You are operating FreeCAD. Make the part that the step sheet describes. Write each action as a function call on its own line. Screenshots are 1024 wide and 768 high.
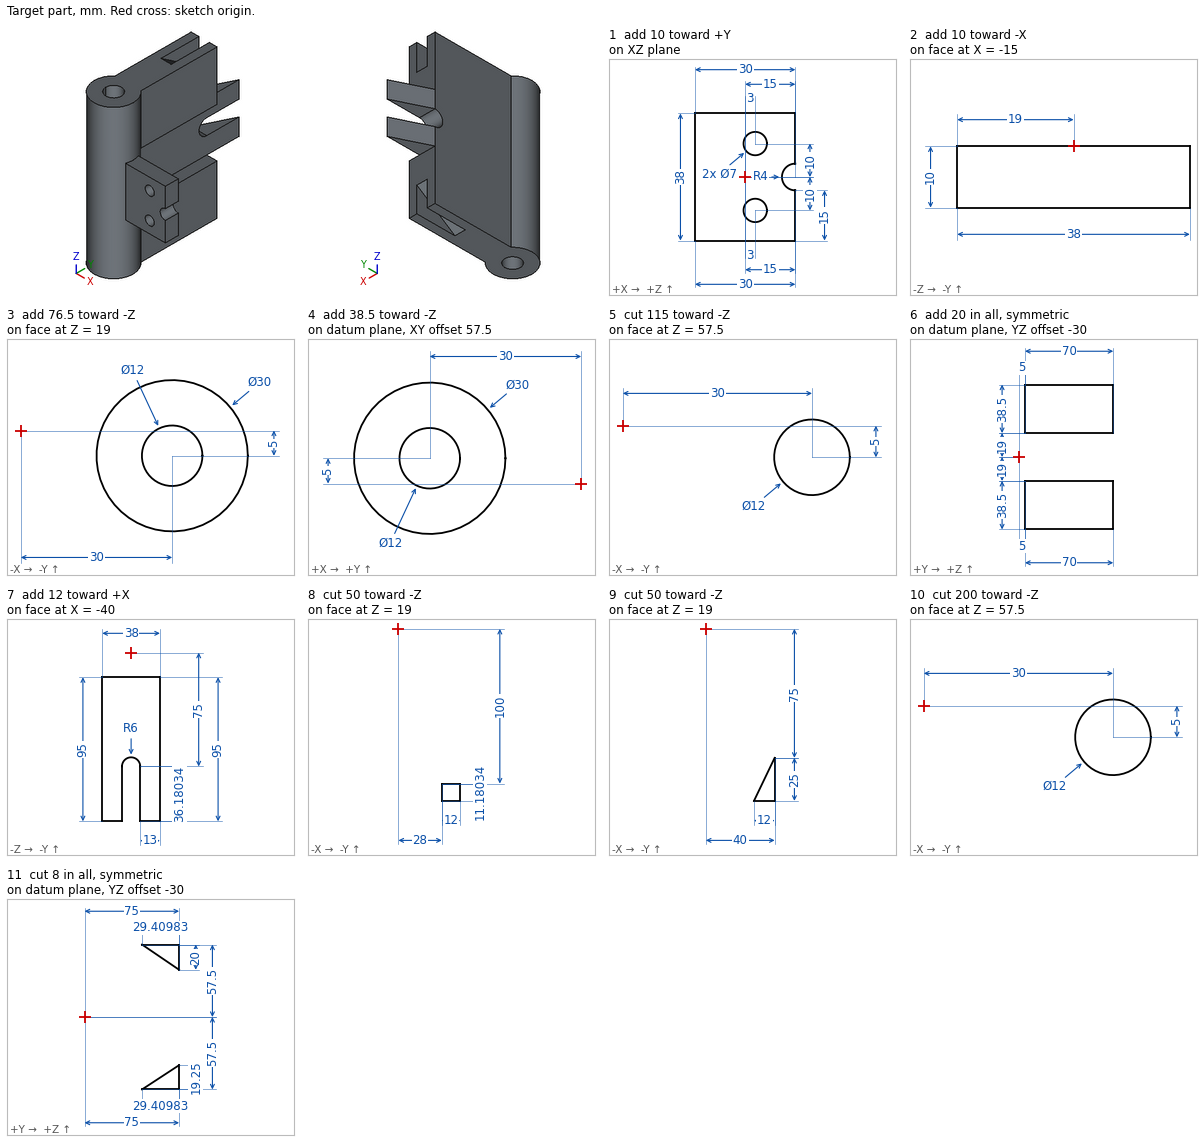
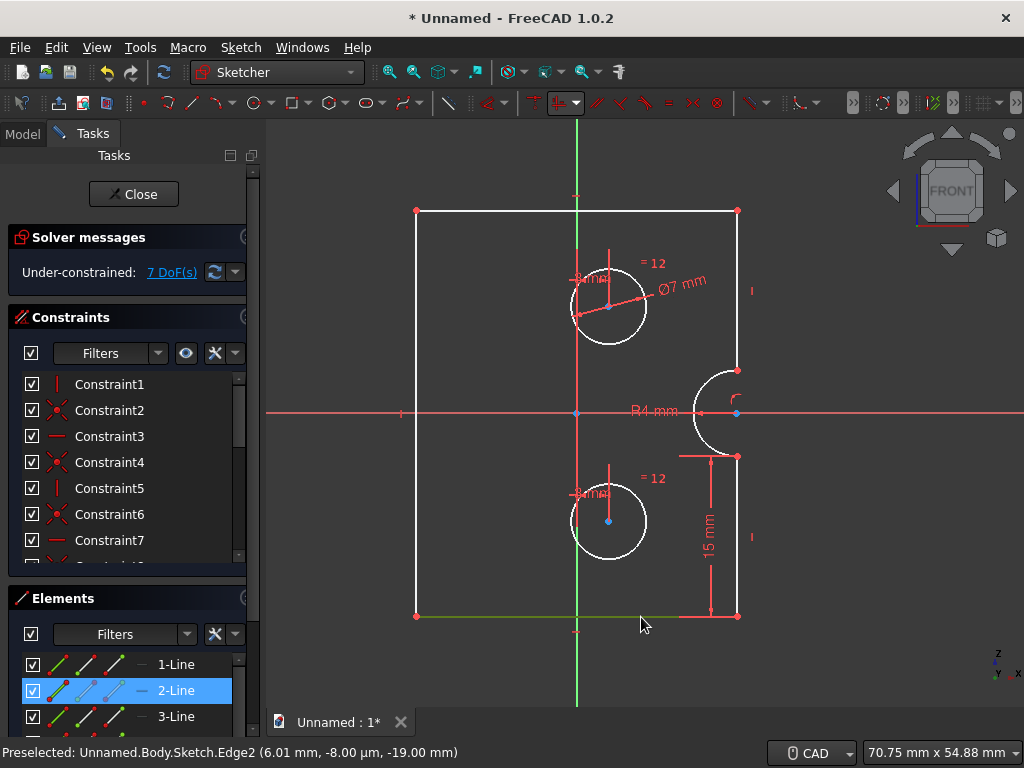
click(506, 104)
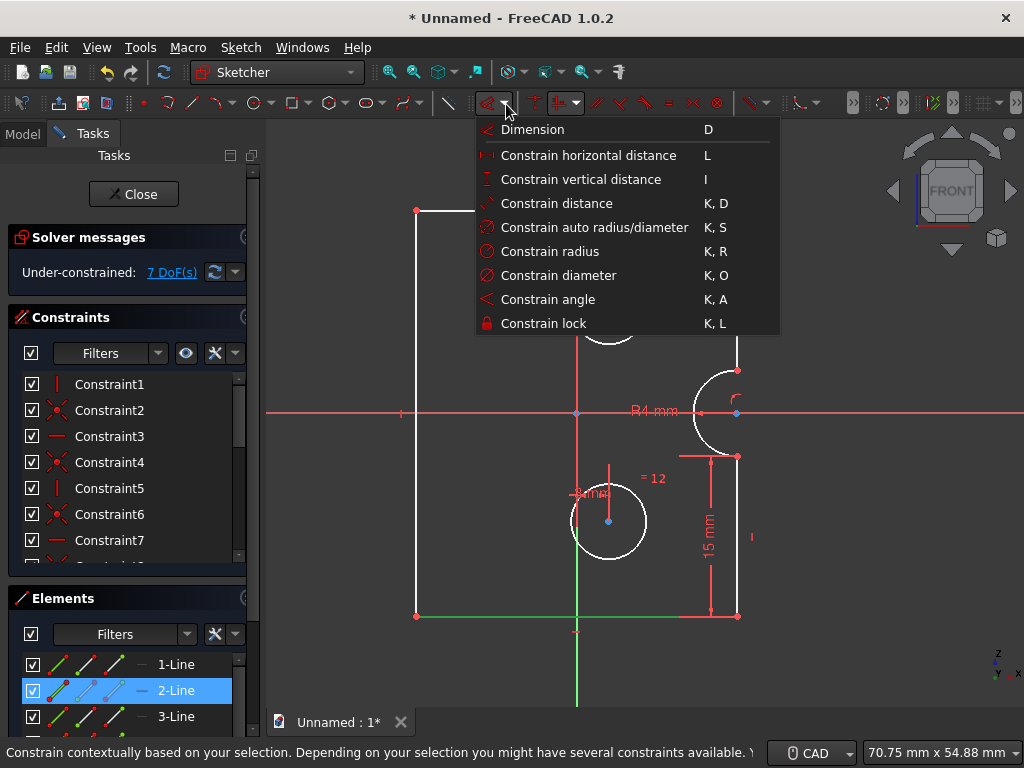
click(628, 155)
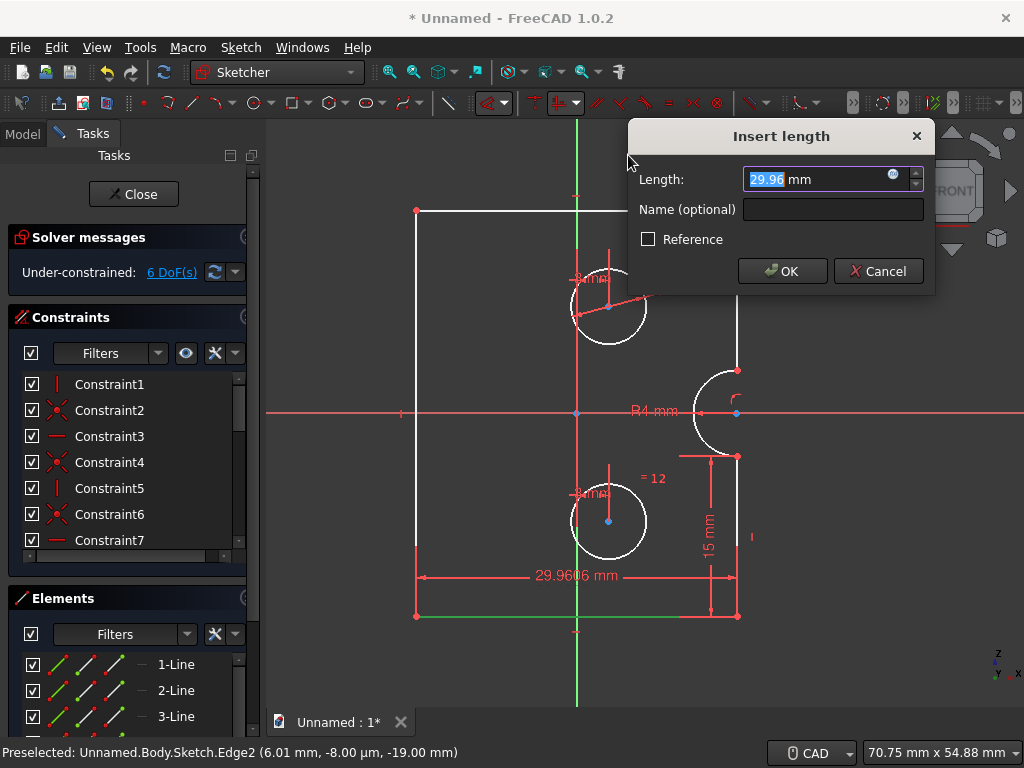
text(30)
key(Return)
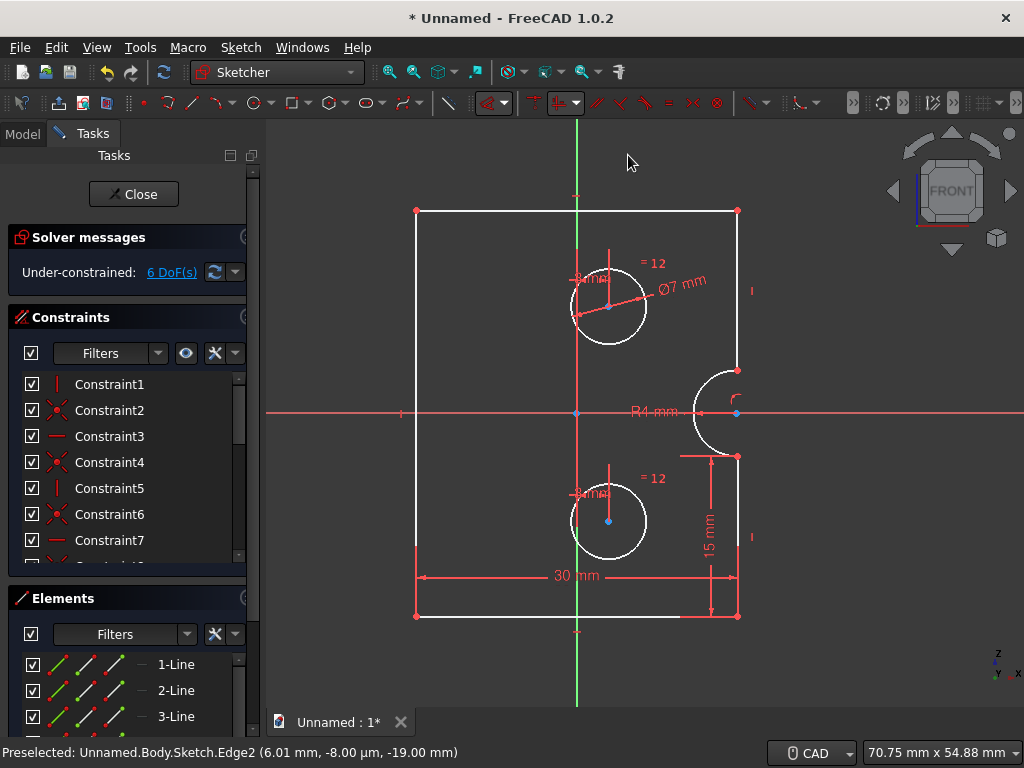
click(416, 495)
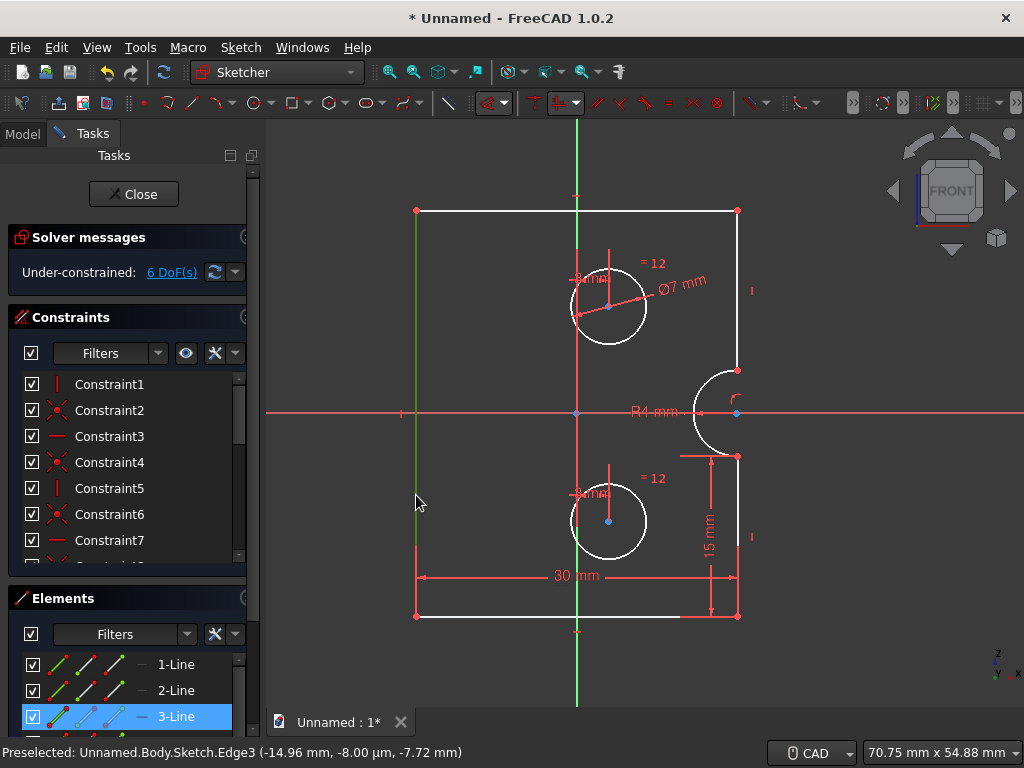
click(506, 104)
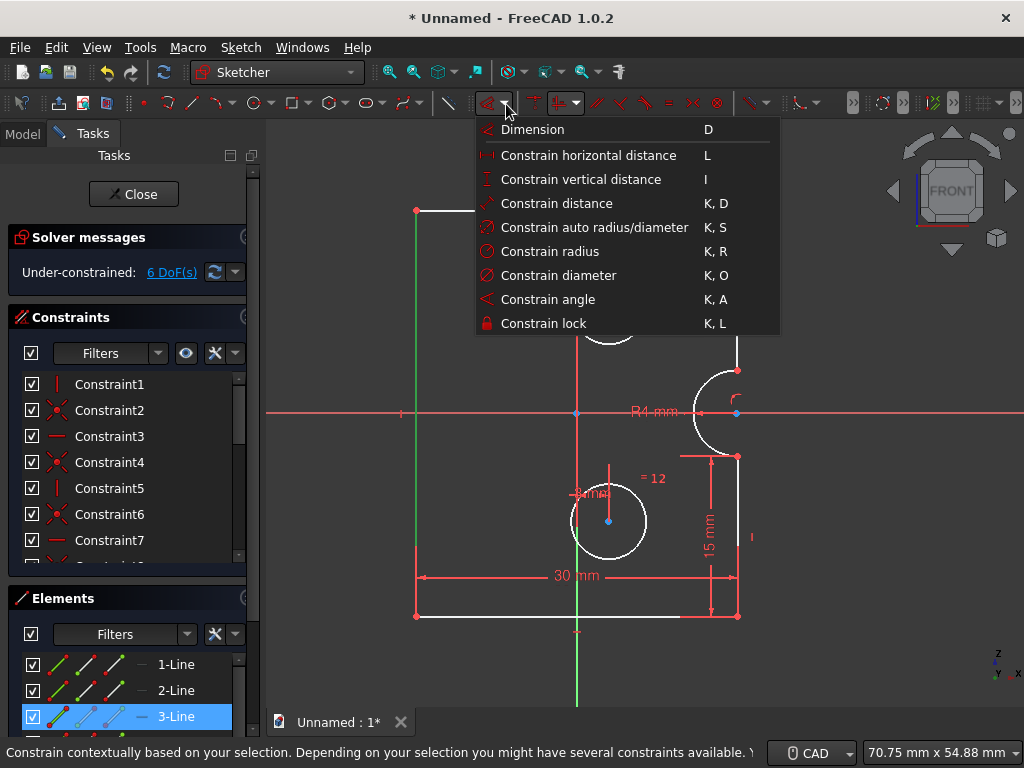
click(628, 179)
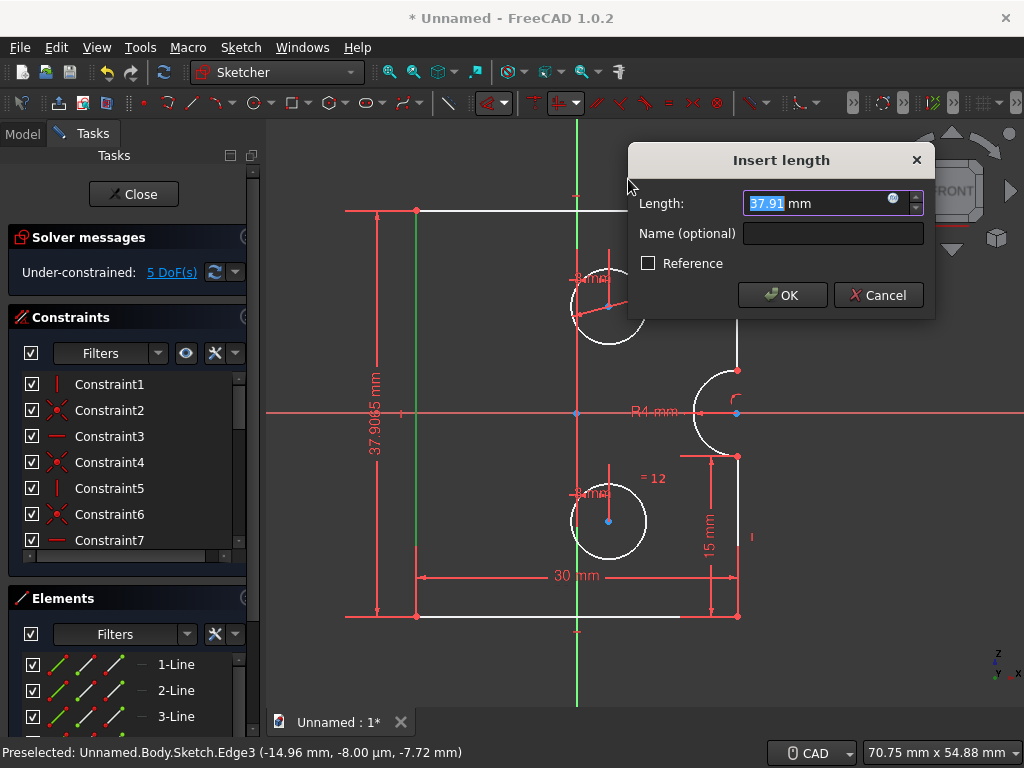
text(38)
key(Return)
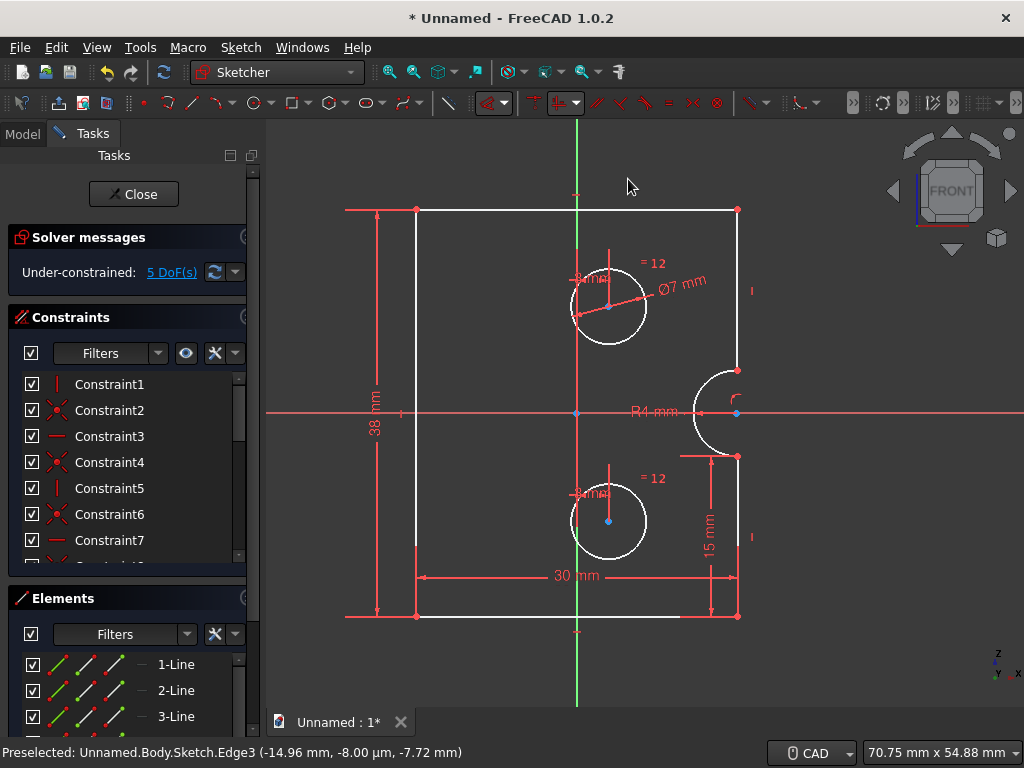
click(513, 210)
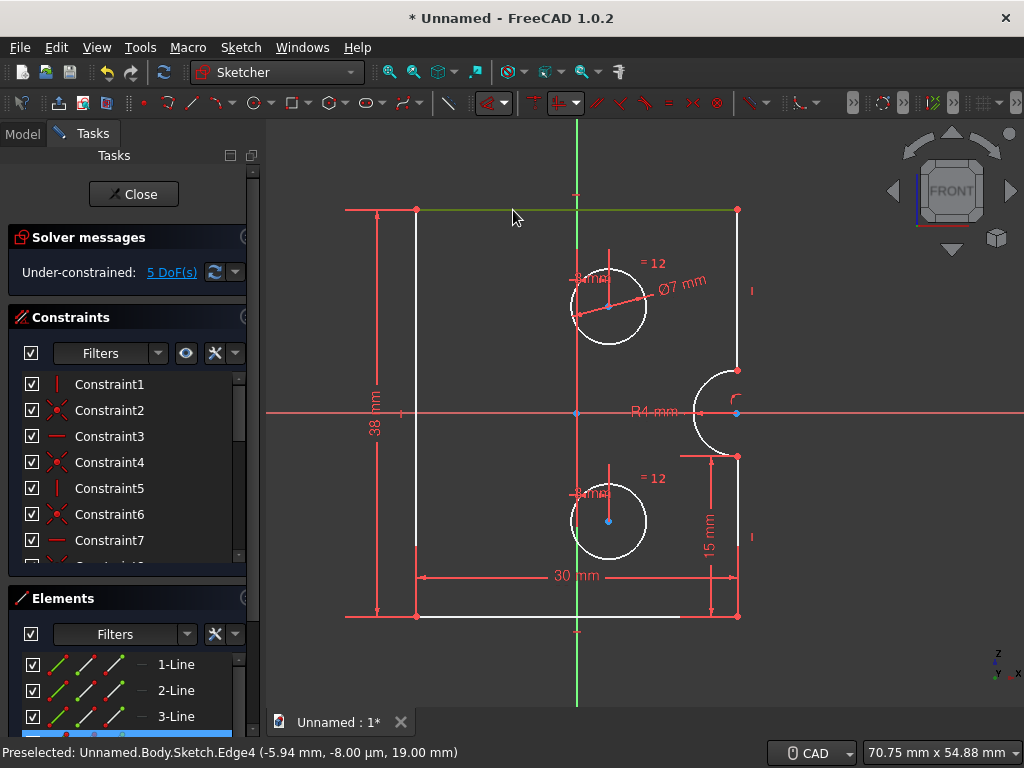
click(506, 104)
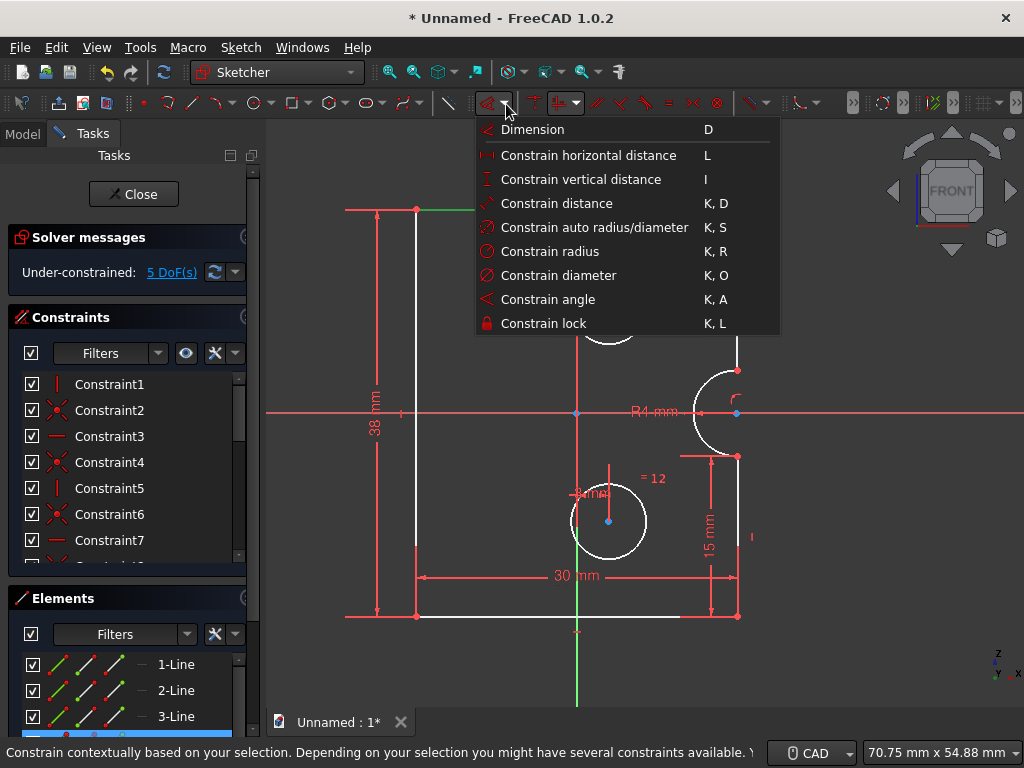
click(628, 155)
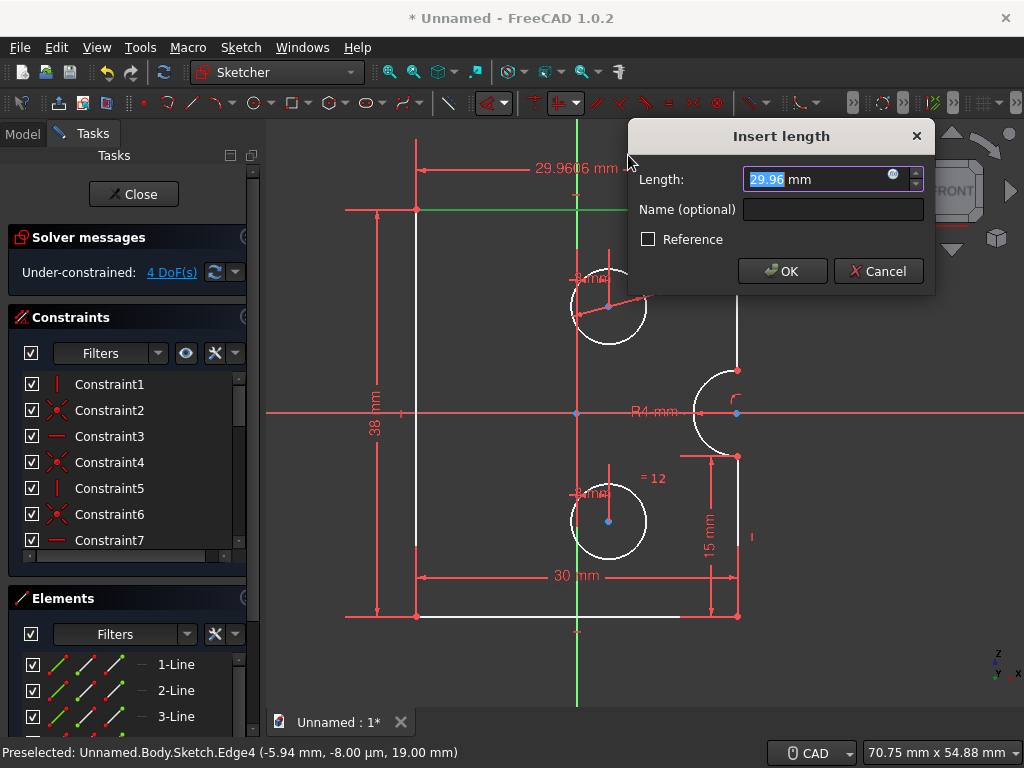
text(30)
key(Return)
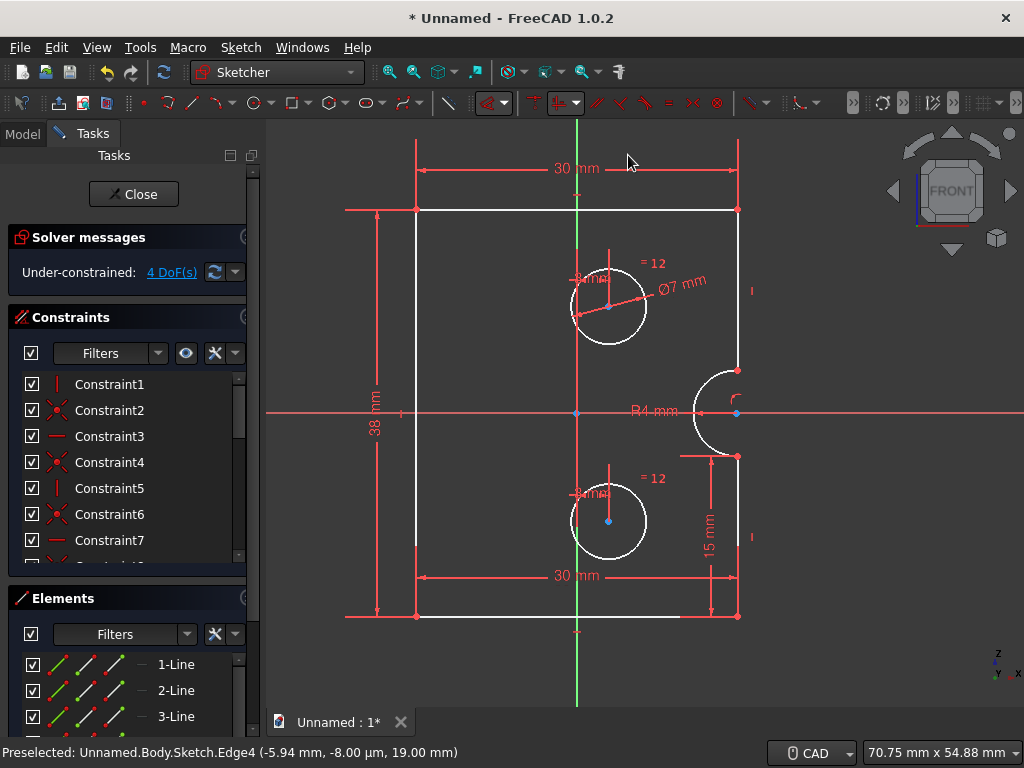
click(609, 307)